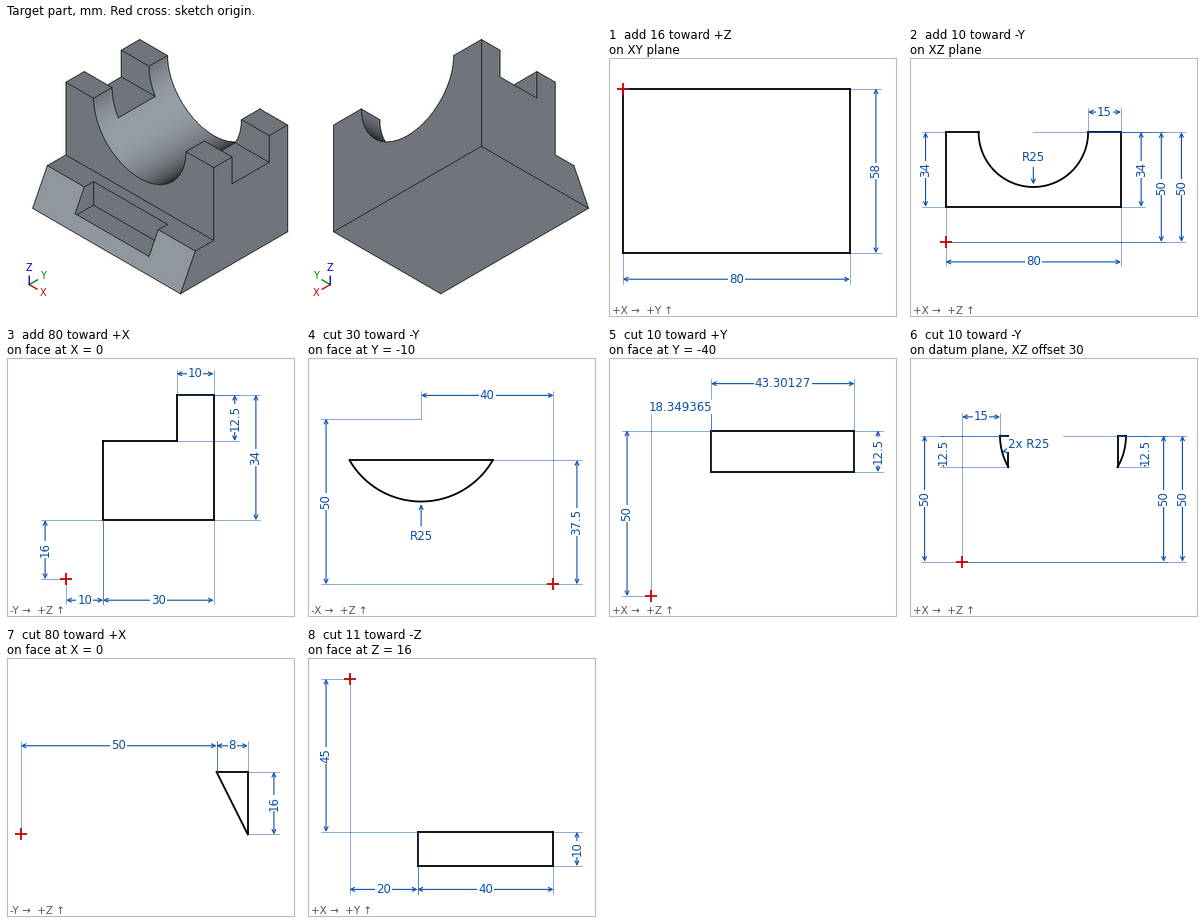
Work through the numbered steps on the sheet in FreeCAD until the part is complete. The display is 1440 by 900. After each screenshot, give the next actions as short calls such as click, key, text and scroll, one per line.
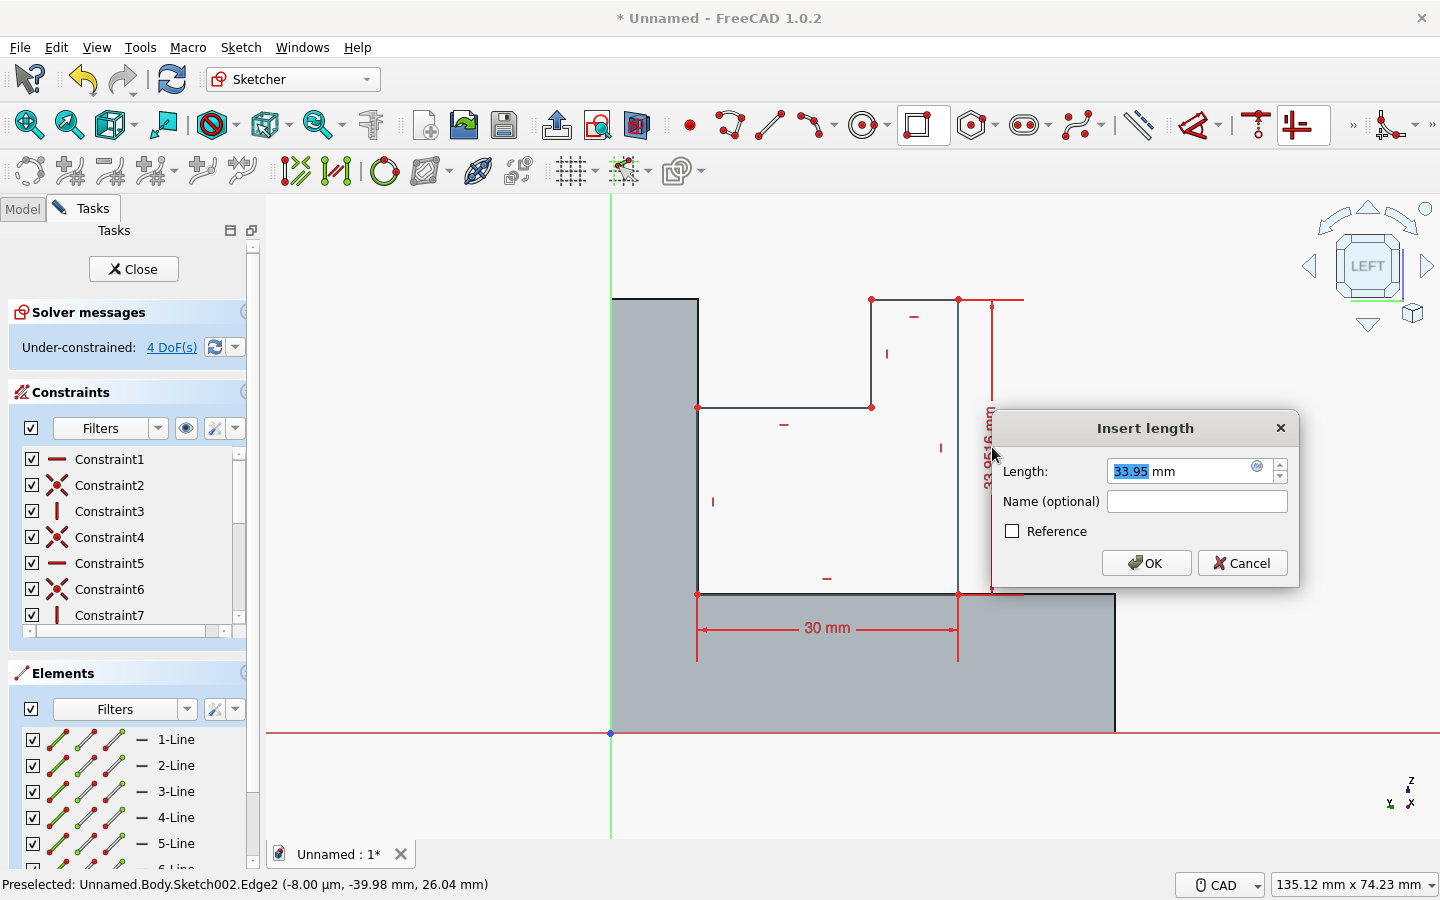
text(34)
key(Return)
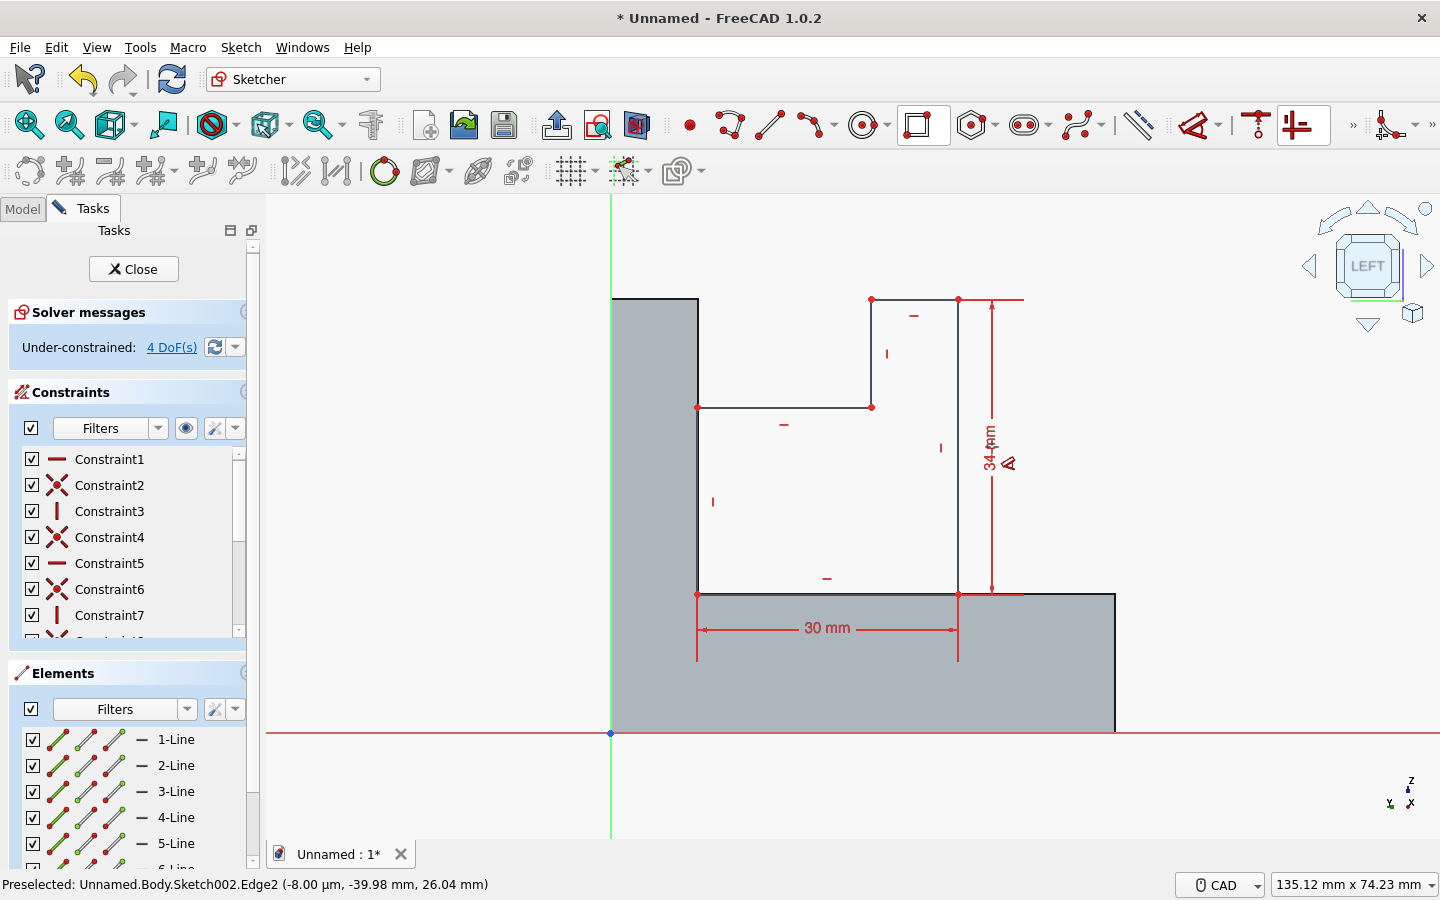
click(932, 300)
click(915, 266)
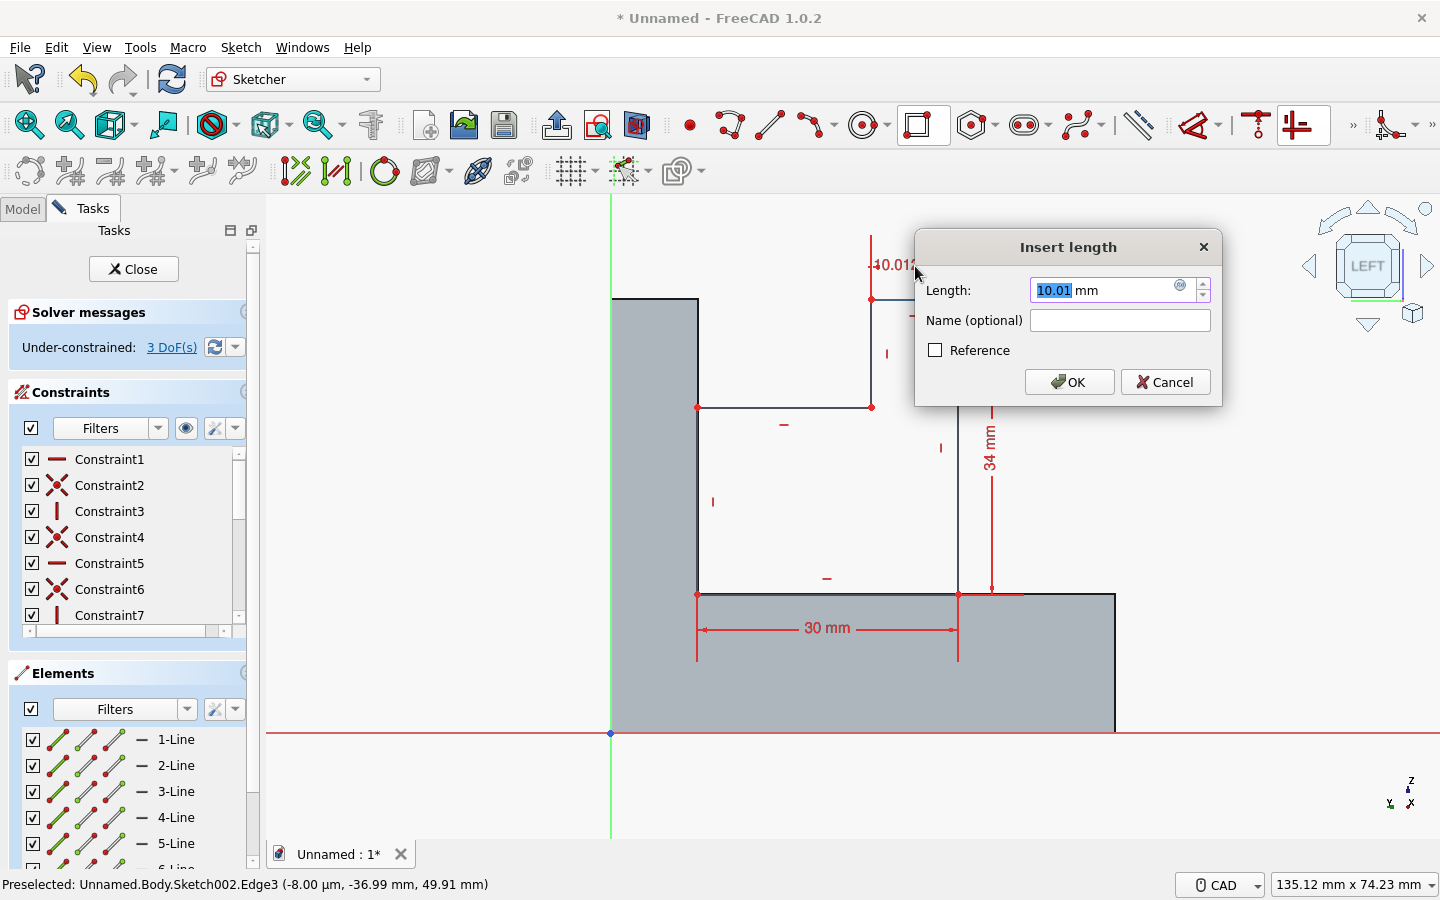
text(10)
key(Return)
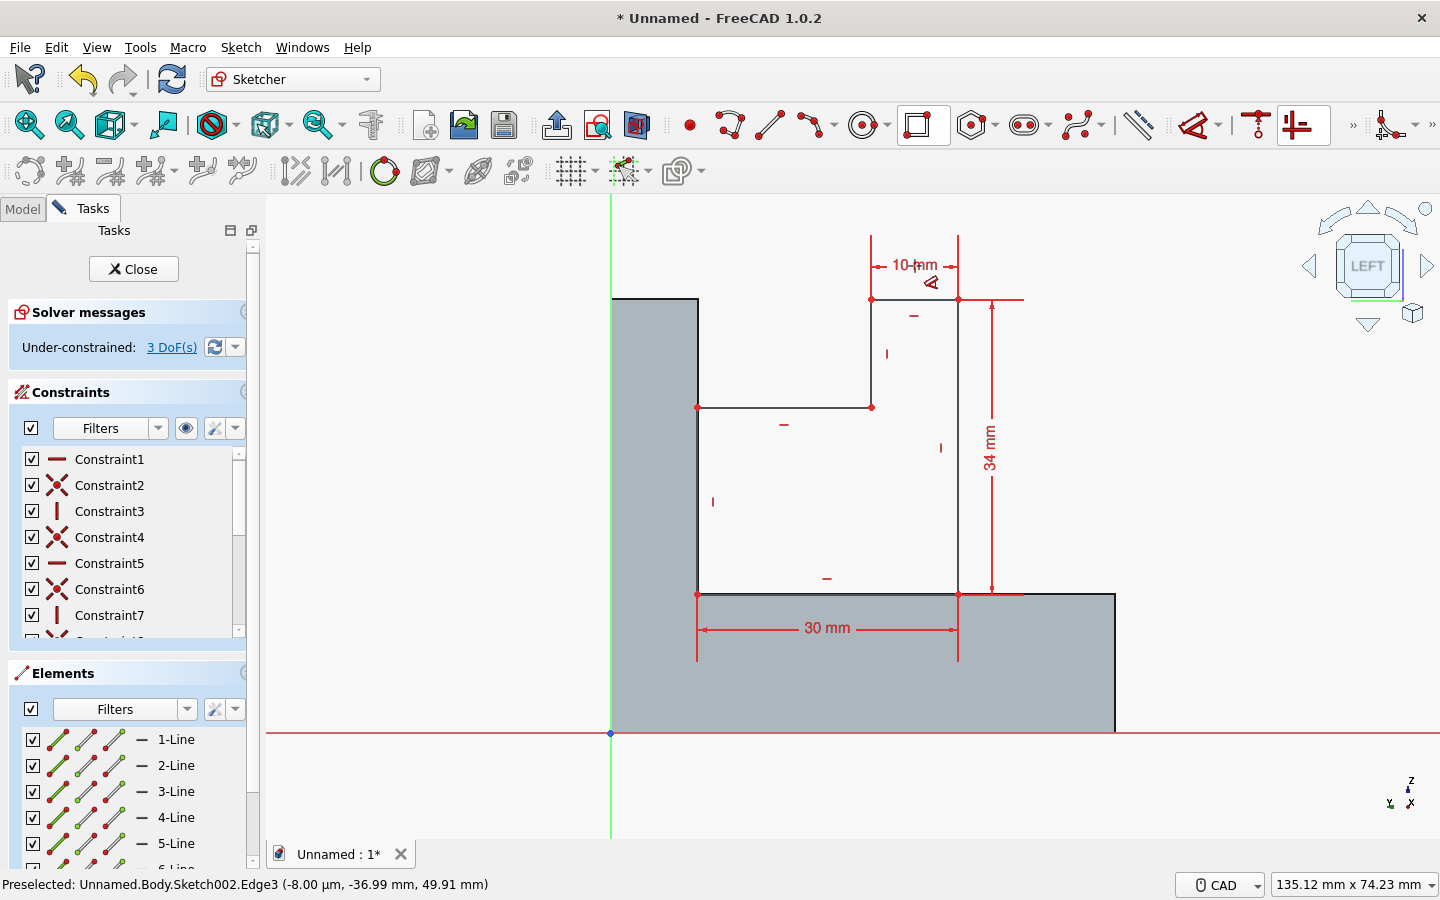
click(697, 595)
click(654, 767)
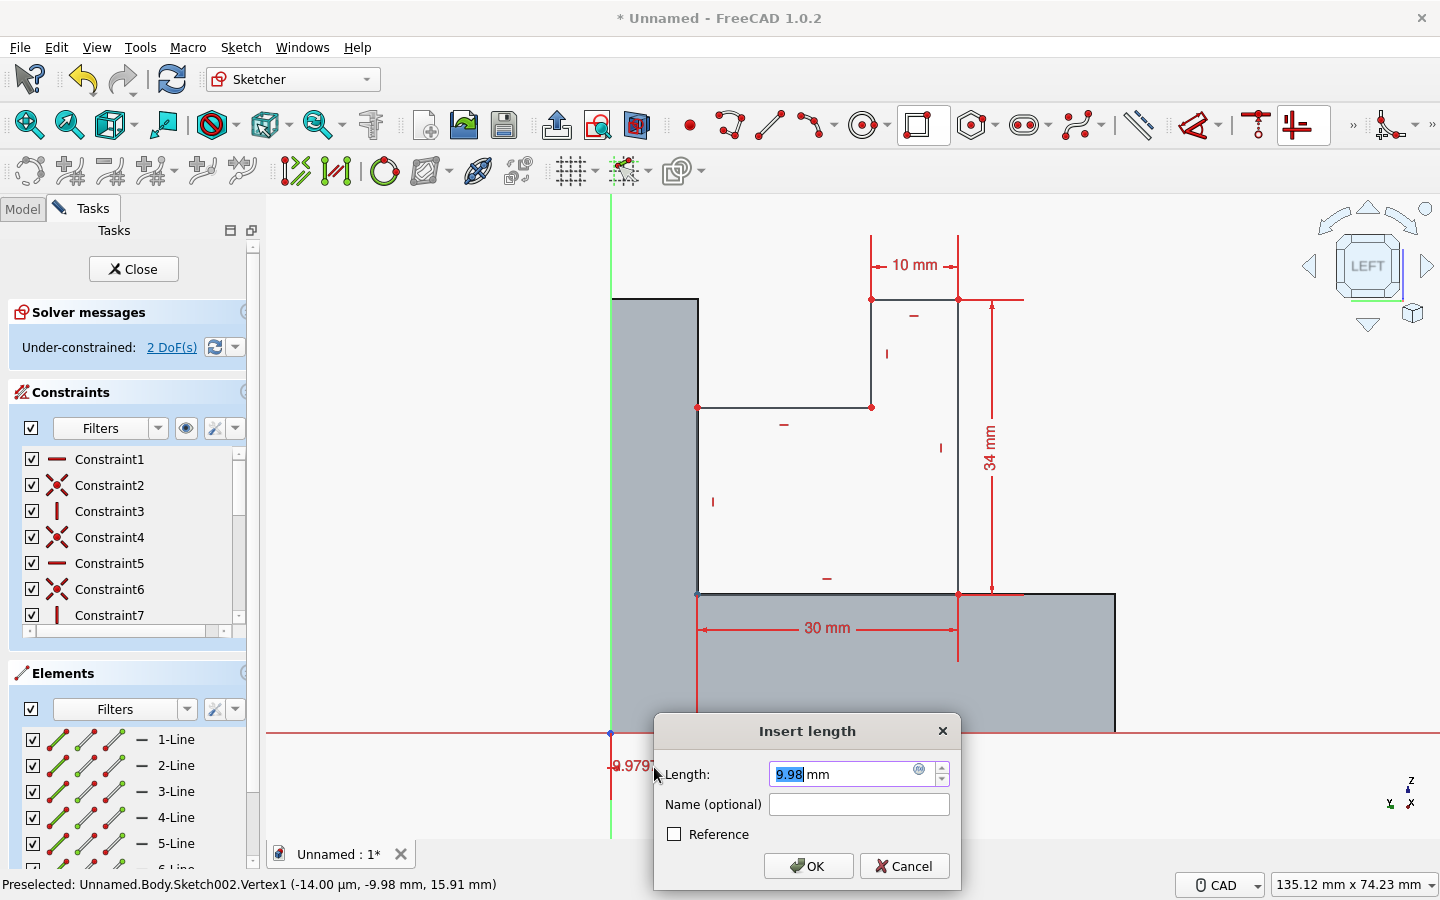
text(10)
key(Return)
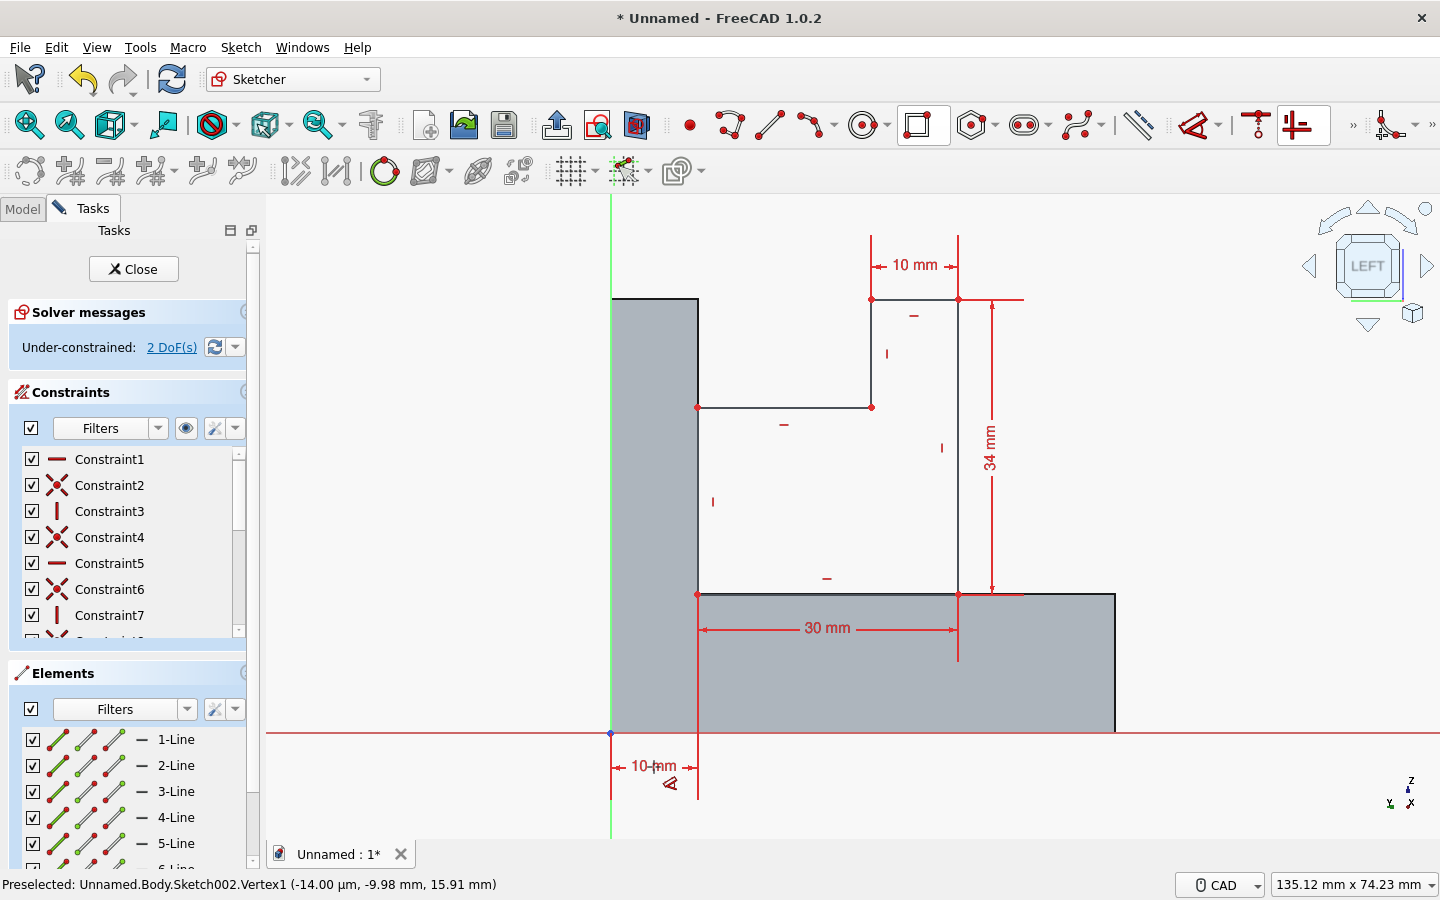
click(698, 595)
click(577, 664)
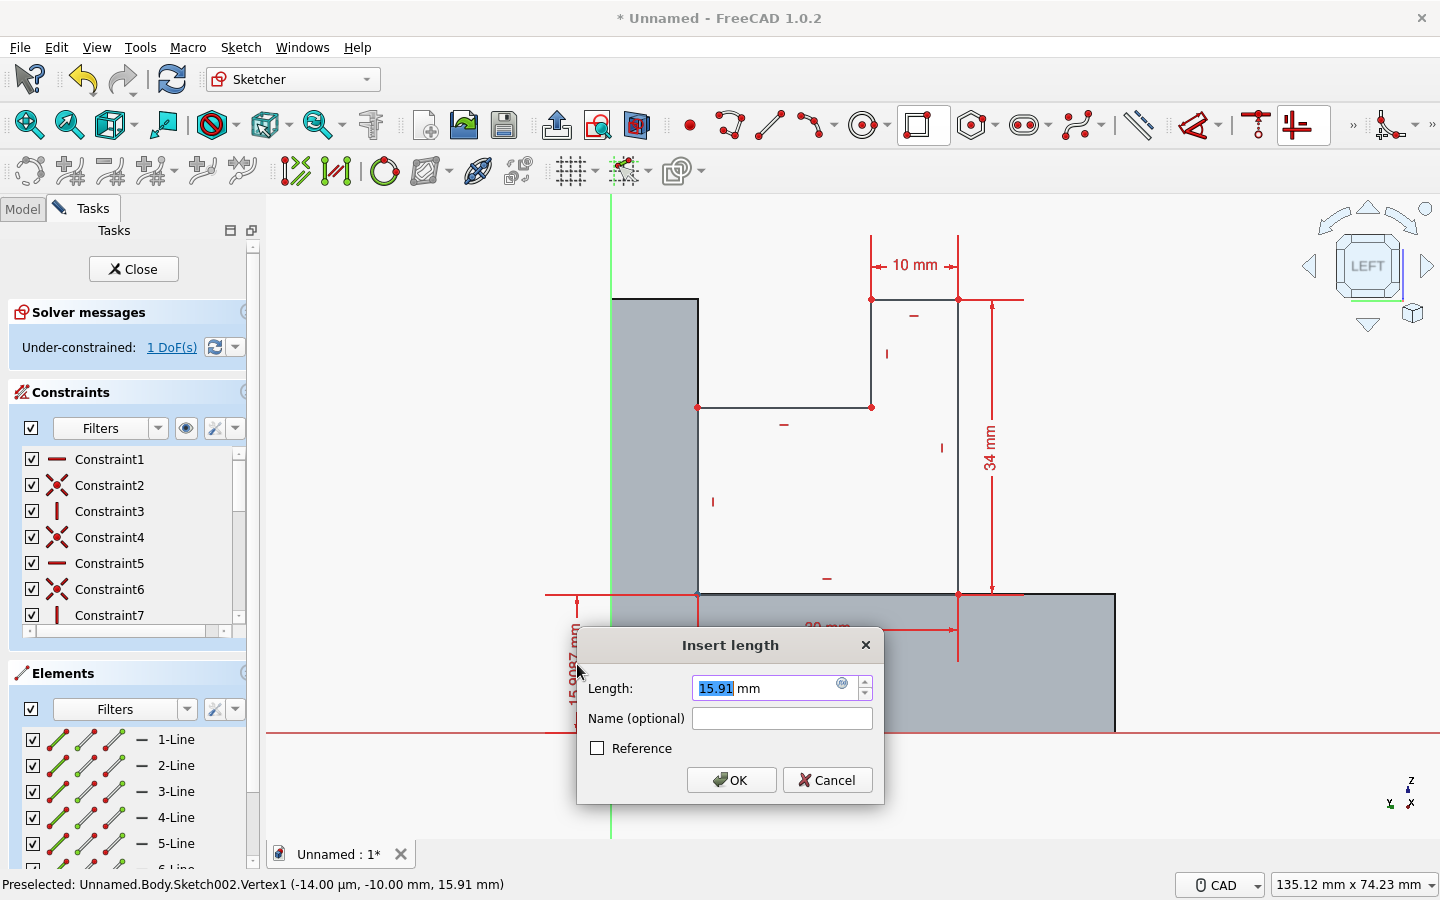
text(16)
key(Return)